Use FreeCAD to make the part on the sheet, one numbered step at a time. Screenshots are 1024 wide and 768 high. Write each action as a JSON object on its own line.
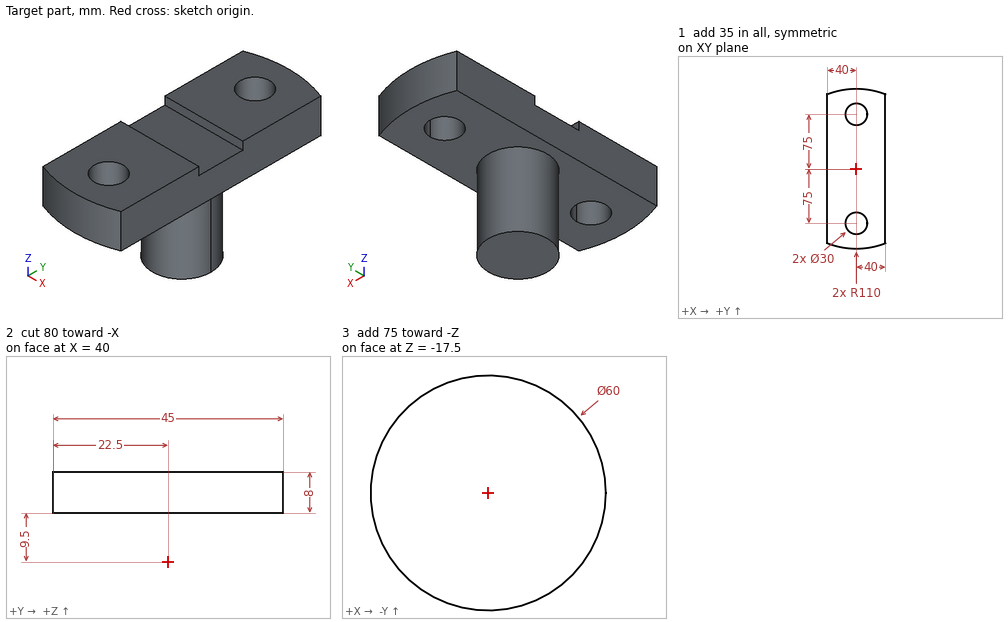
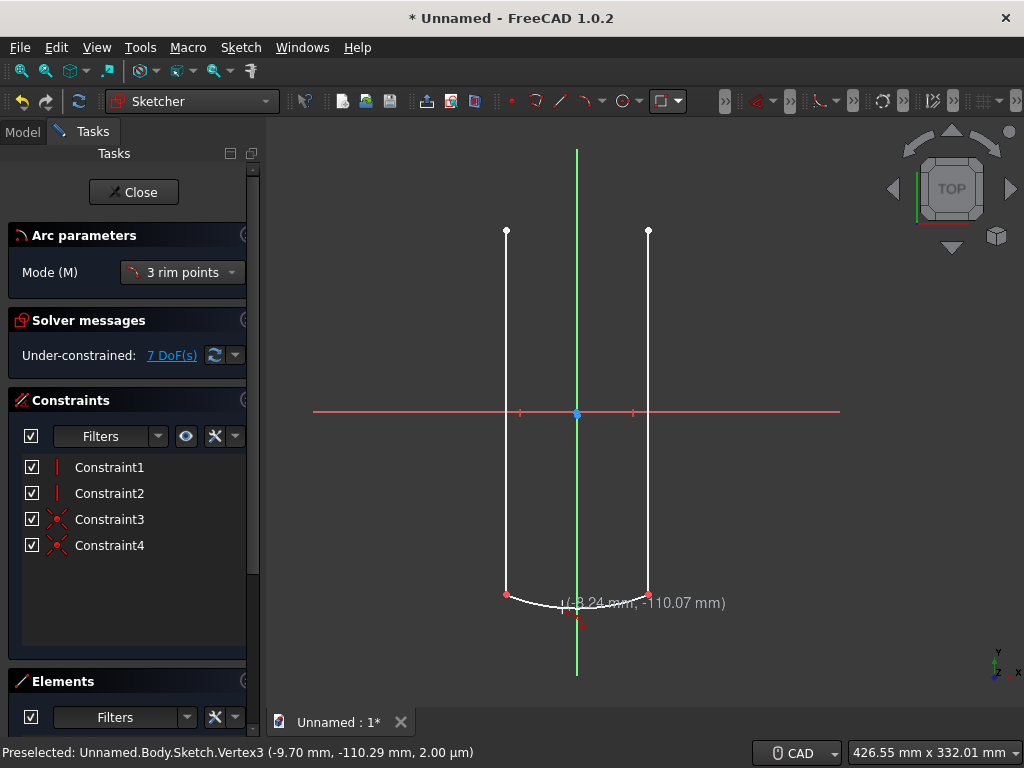
{"action": "left_click", "coordinate": [648, 231]}
{"action": "left_click", "coordinate": [506, 231]}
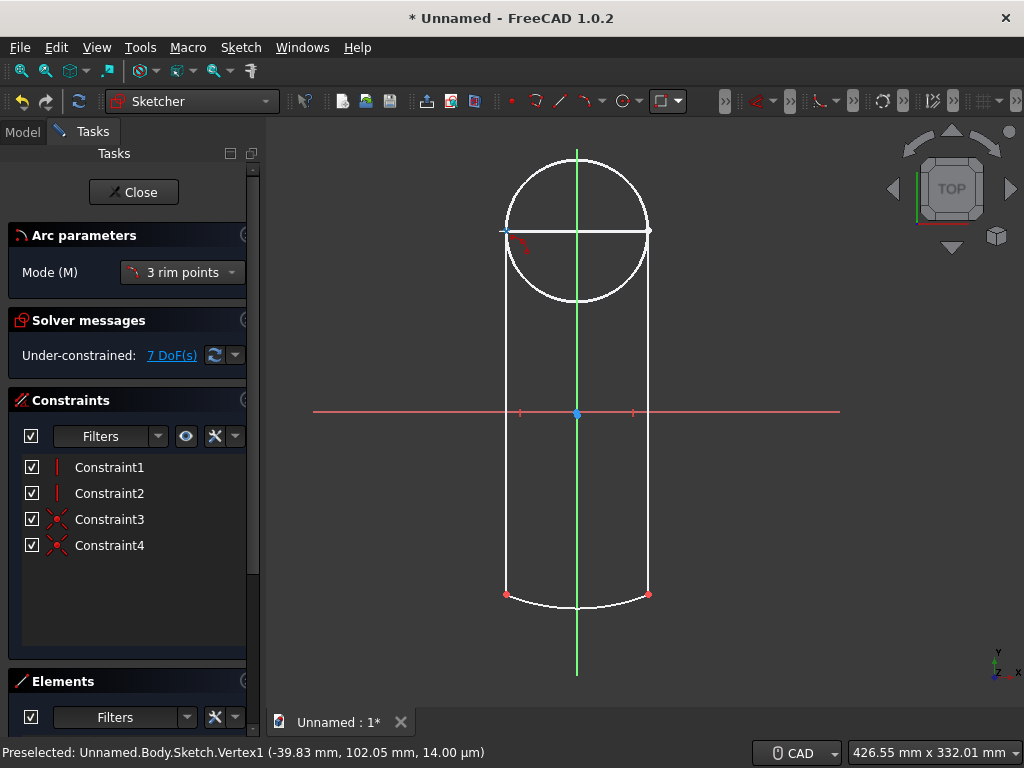
{"action": "scroll", "coordinate": [591, 217], "scroll_direction": "up", "scroll_amount": 2}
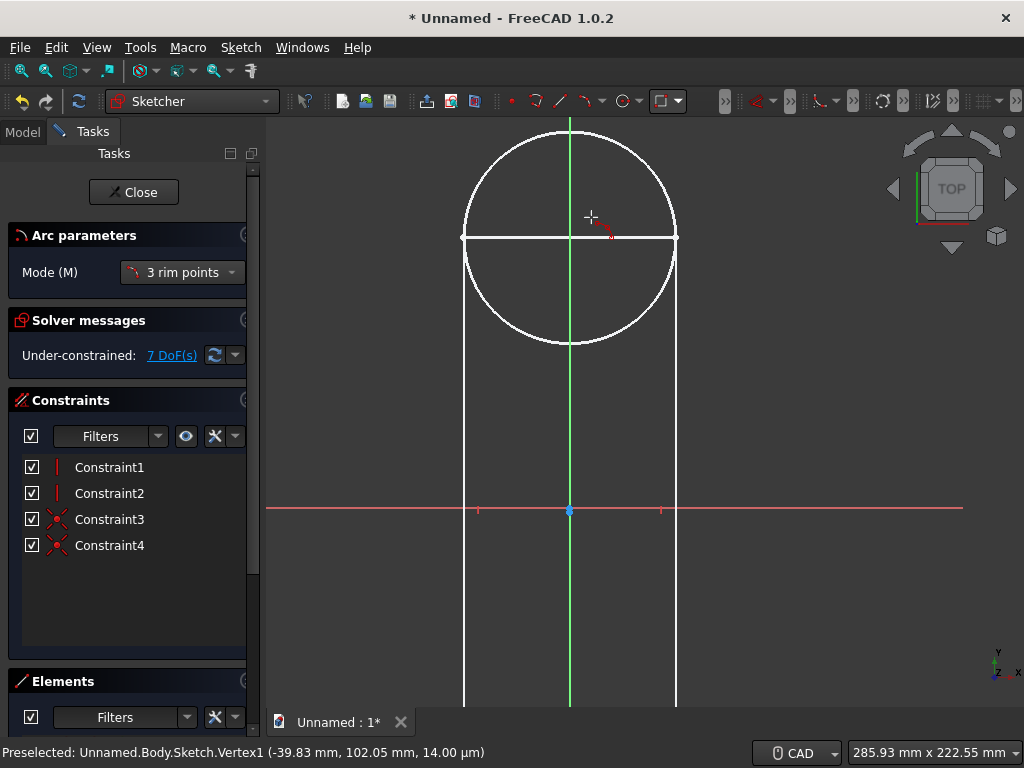
{"action": "left_click", "coordinate": [591, 218]}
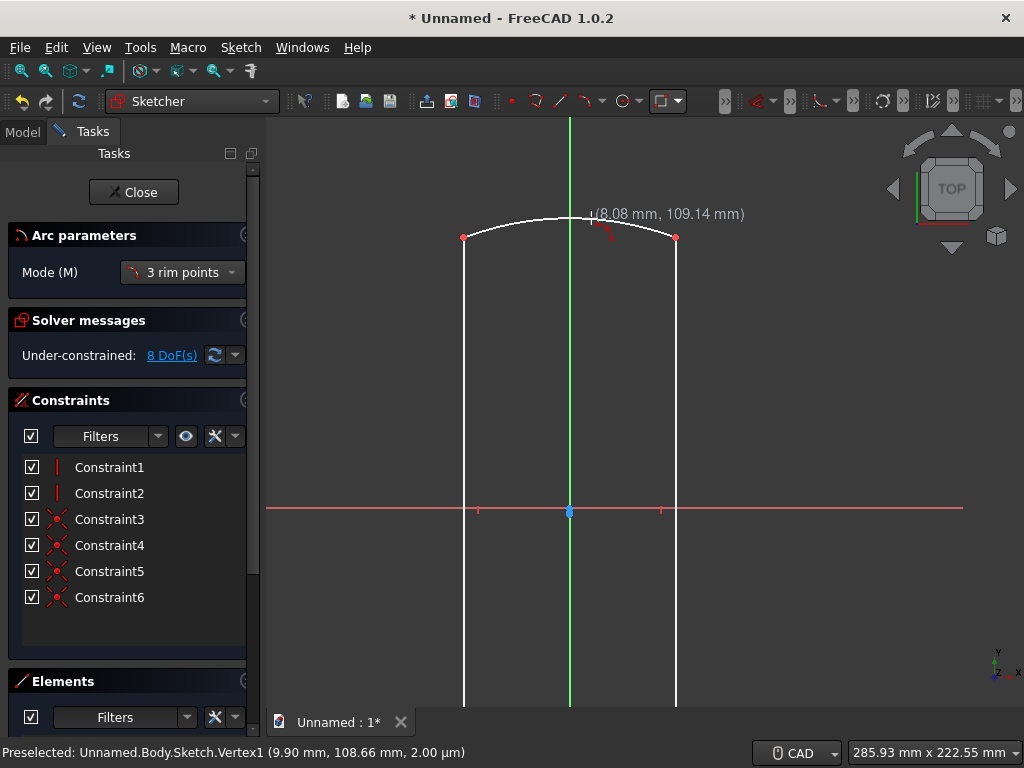
{"action": "key", "text": "g c"}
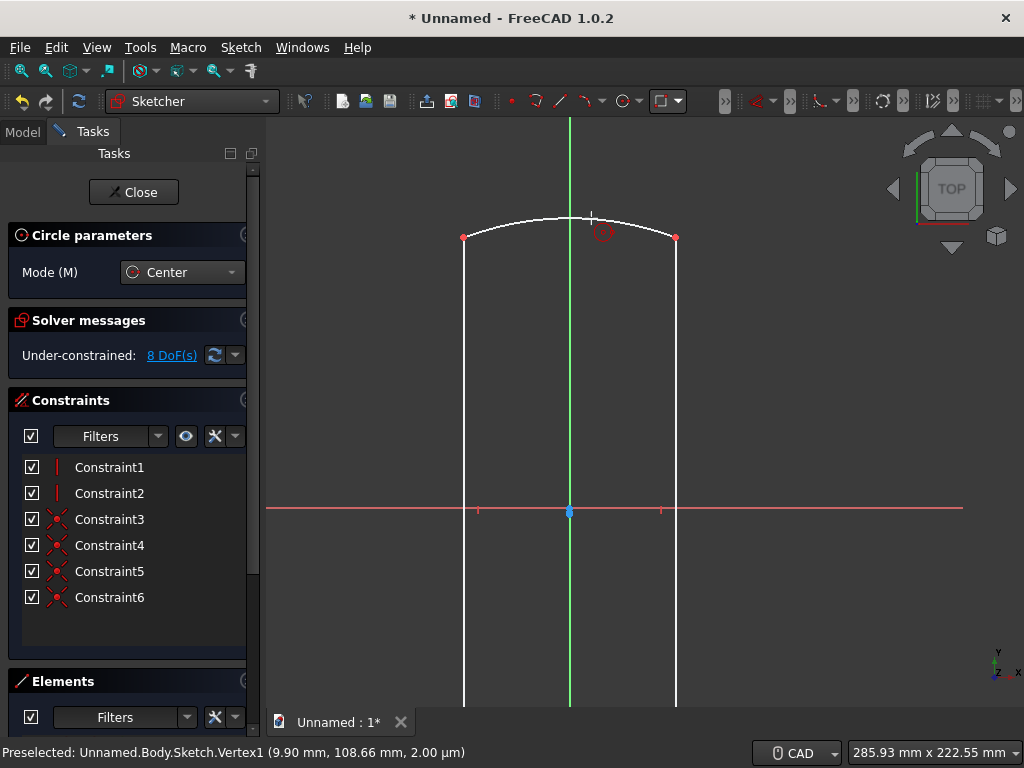
{"action": "scroll", "coordinate": [591, 216], "scroll_direction": "down", "scroll_amount": 2}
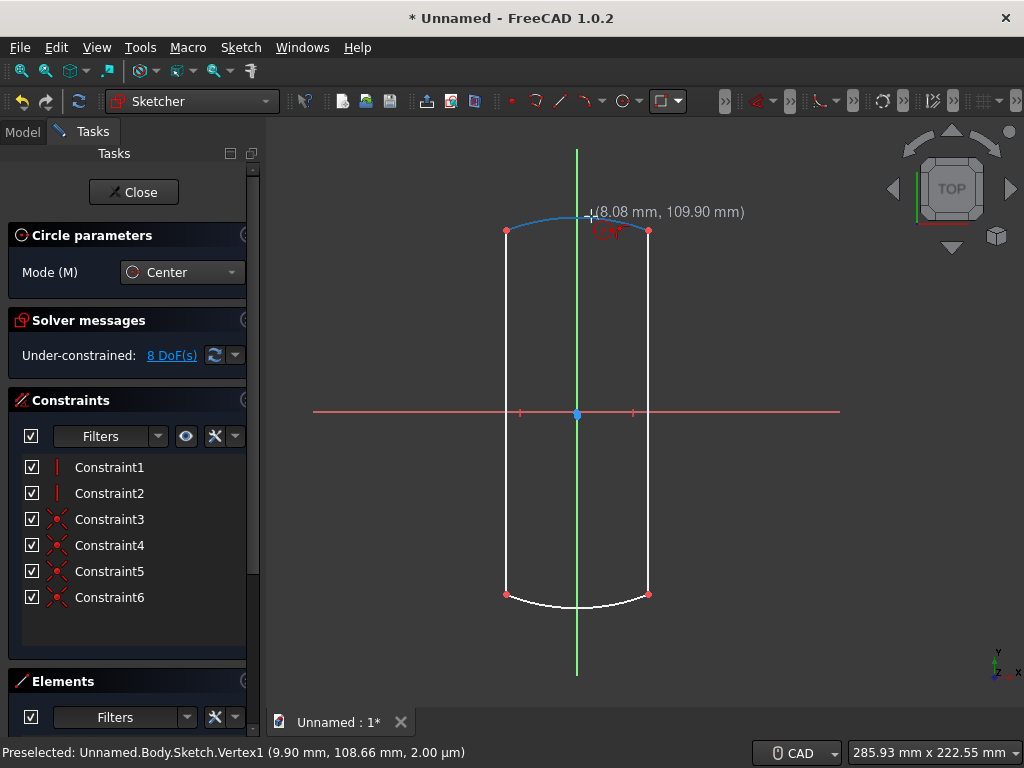
{"action": "left_click", "coordinate": [577, 545]}
{"action": "mouse_move", "coordinate": [596, 526]}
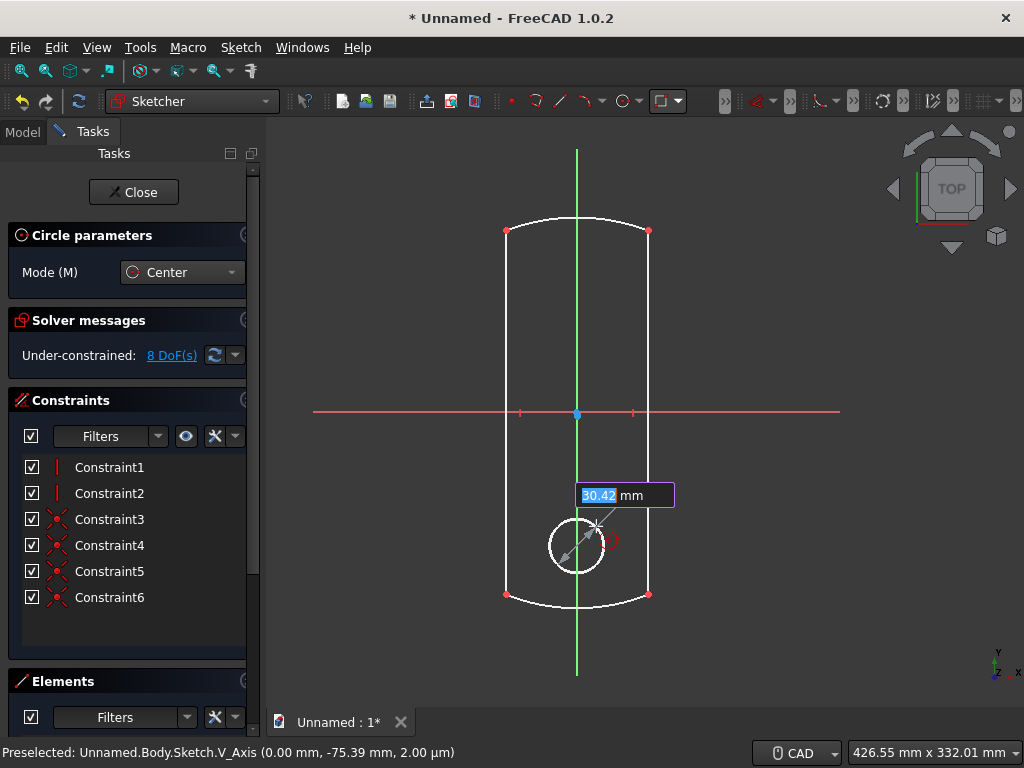
{"action": "type", "text": "30"}
{"action": "key", "text": "Return"}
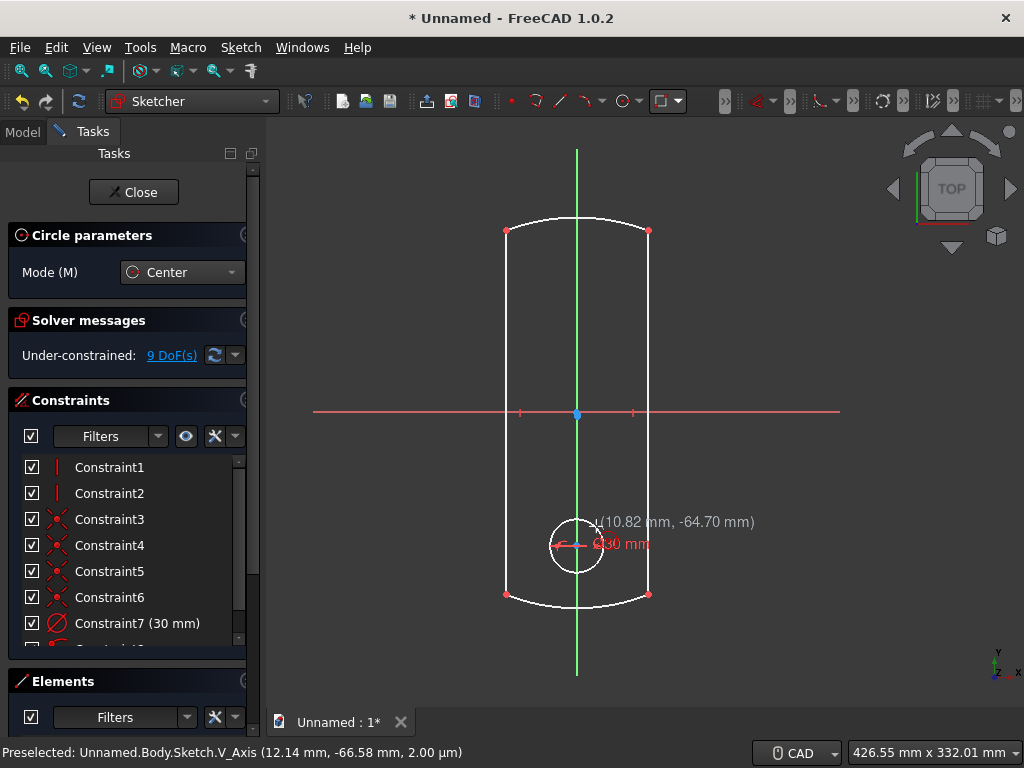
{"action": "left_click", "coordinate": [577, 279]}
{"action": "mouse_move", "coordinate": [596, 260]}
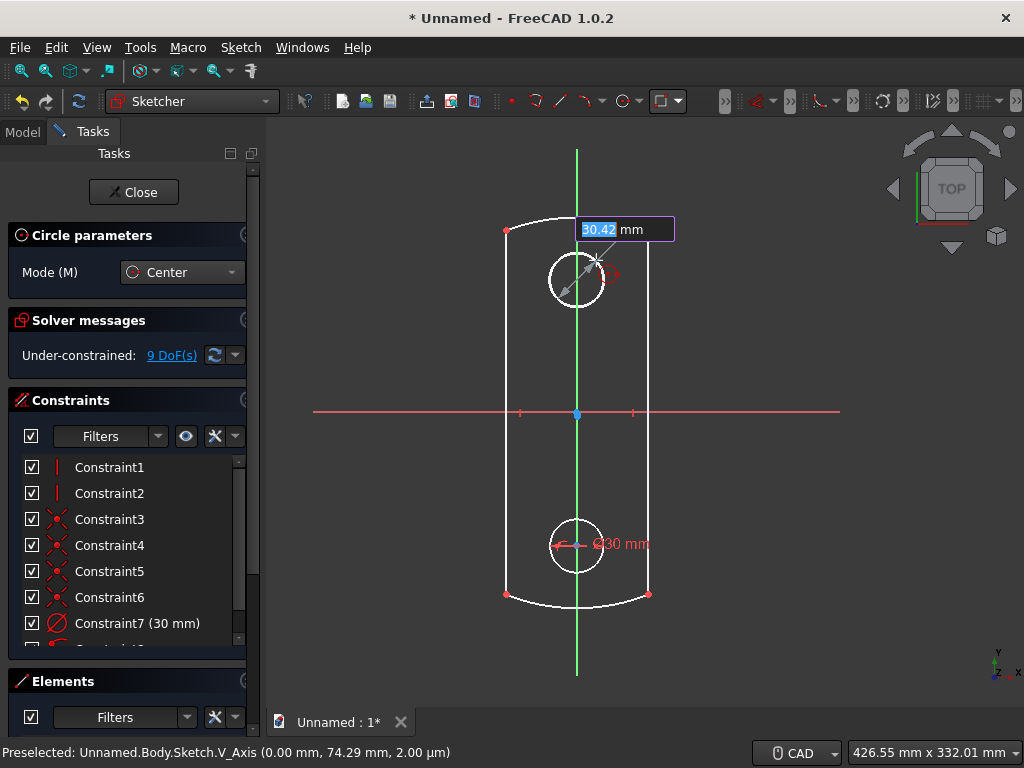
{"action": "type", "text": "30"}
{"action": "key", "text": "Return"}
{"action": "key", "text": "Escape"}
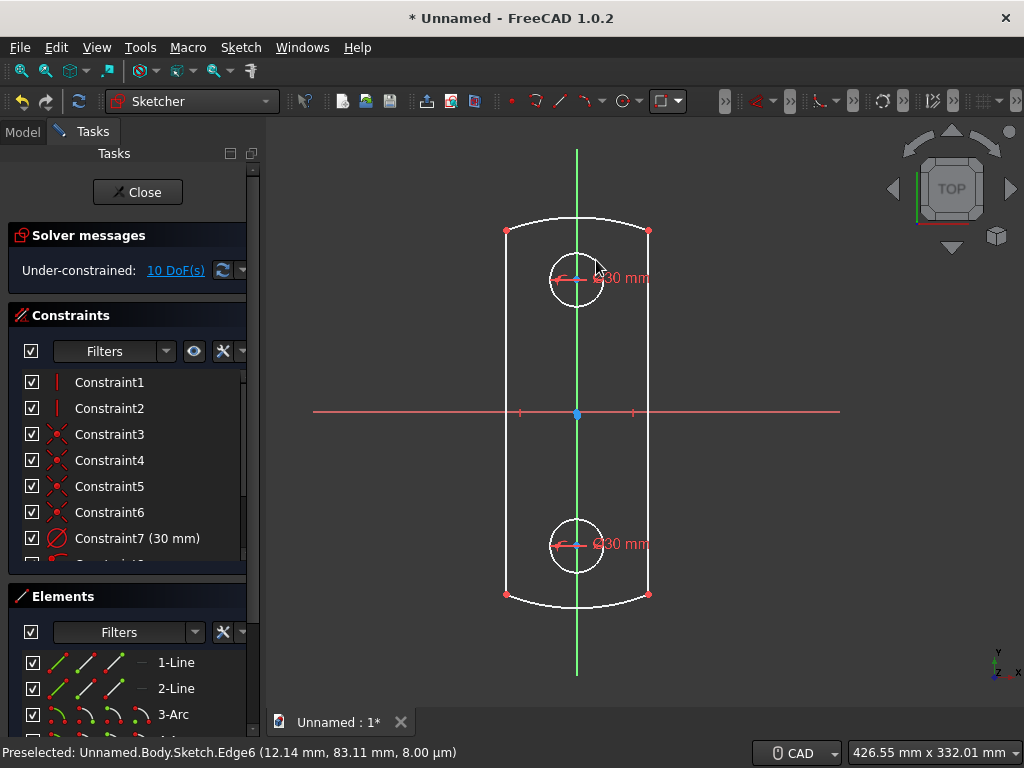
{"action": "left_click", "coordinate": [548, 606]}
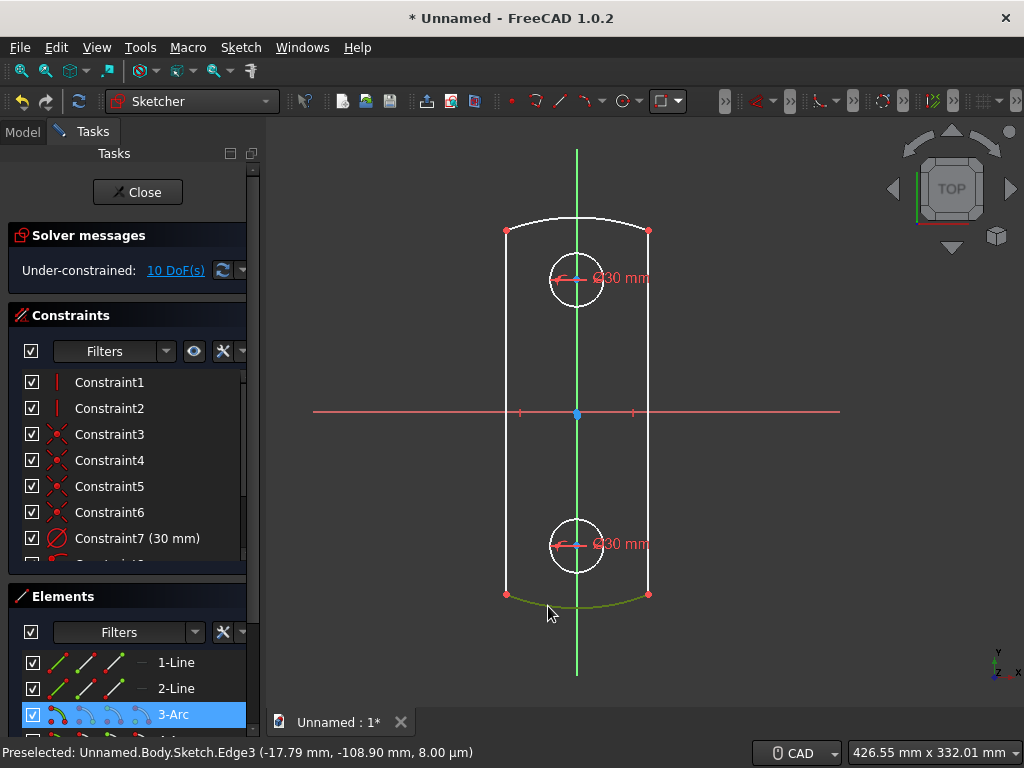
{"action": "left_click", "coordinate": [606, 220]}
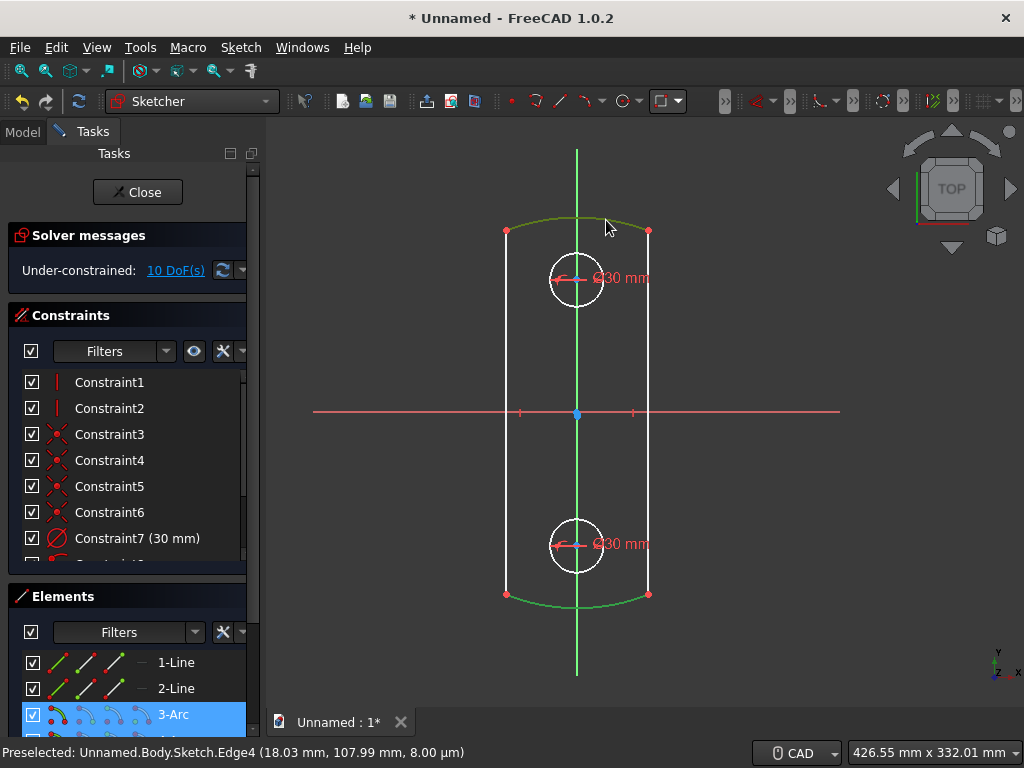
{"action": "key", "text": "c"}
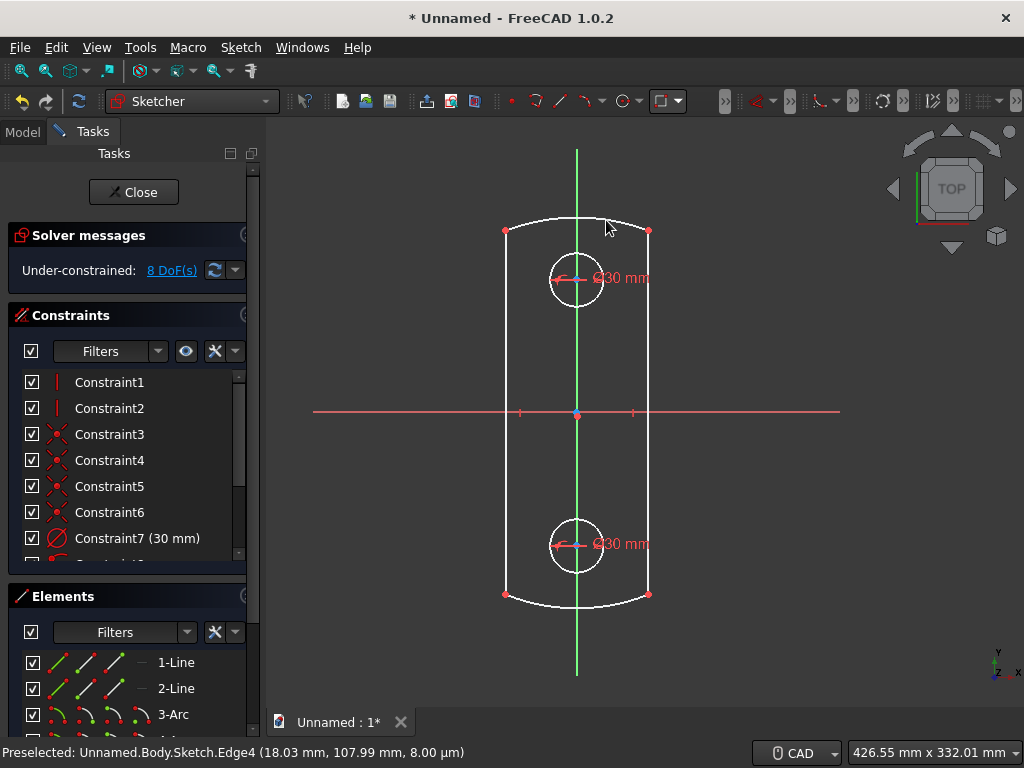
{"action": "scroll", "coordinate": [577, 414], "scroll_direction": "up", "scroll_amount": 2}